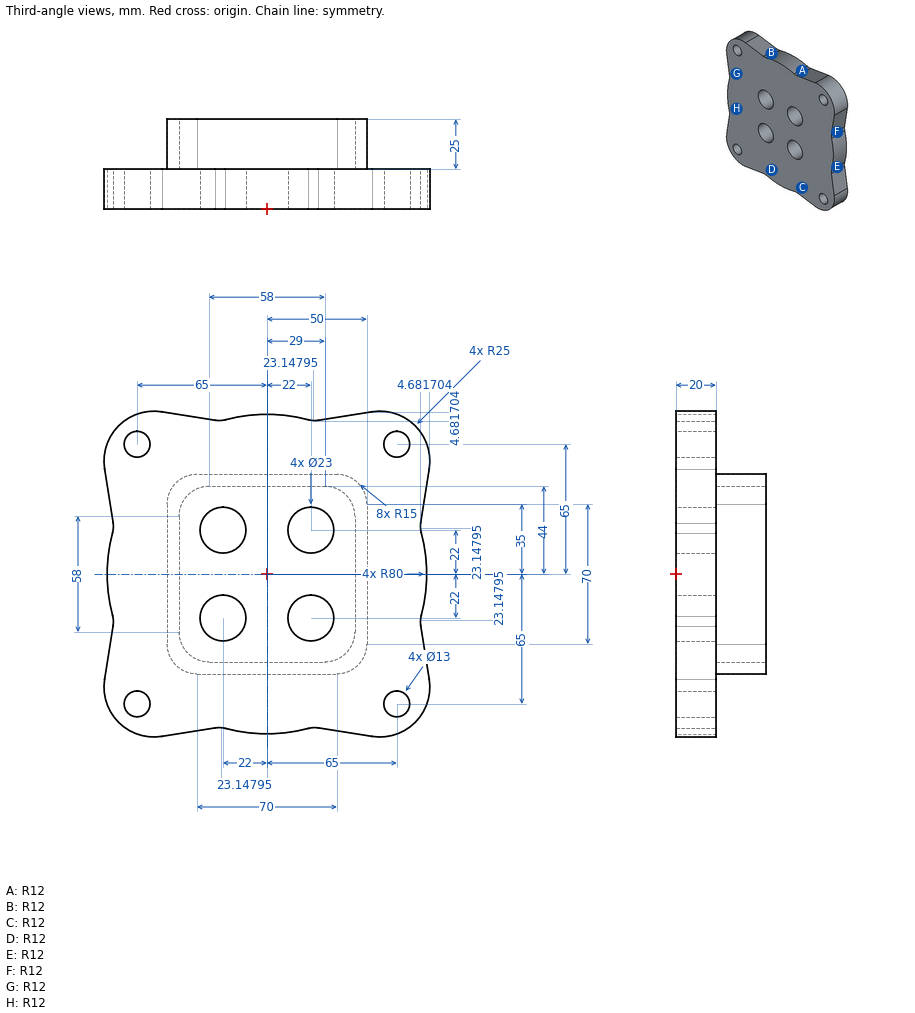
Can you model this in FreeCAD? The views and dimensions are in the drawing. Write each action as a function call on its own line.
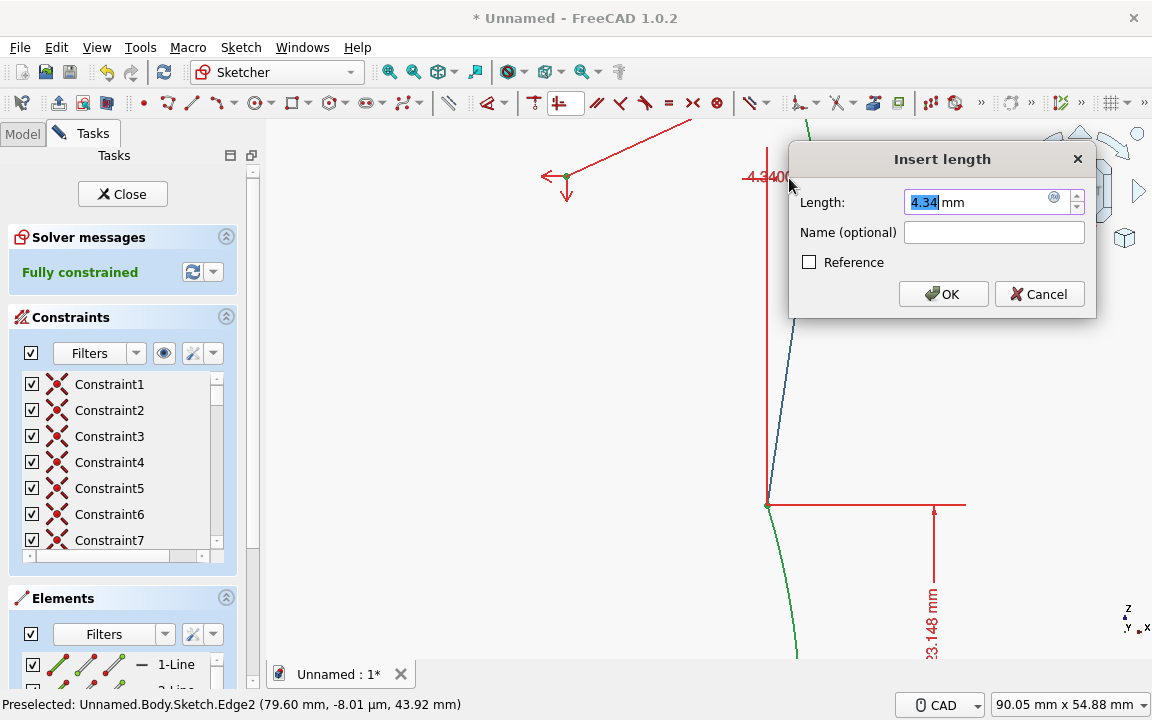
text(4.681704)
key(Return)
key(Escape)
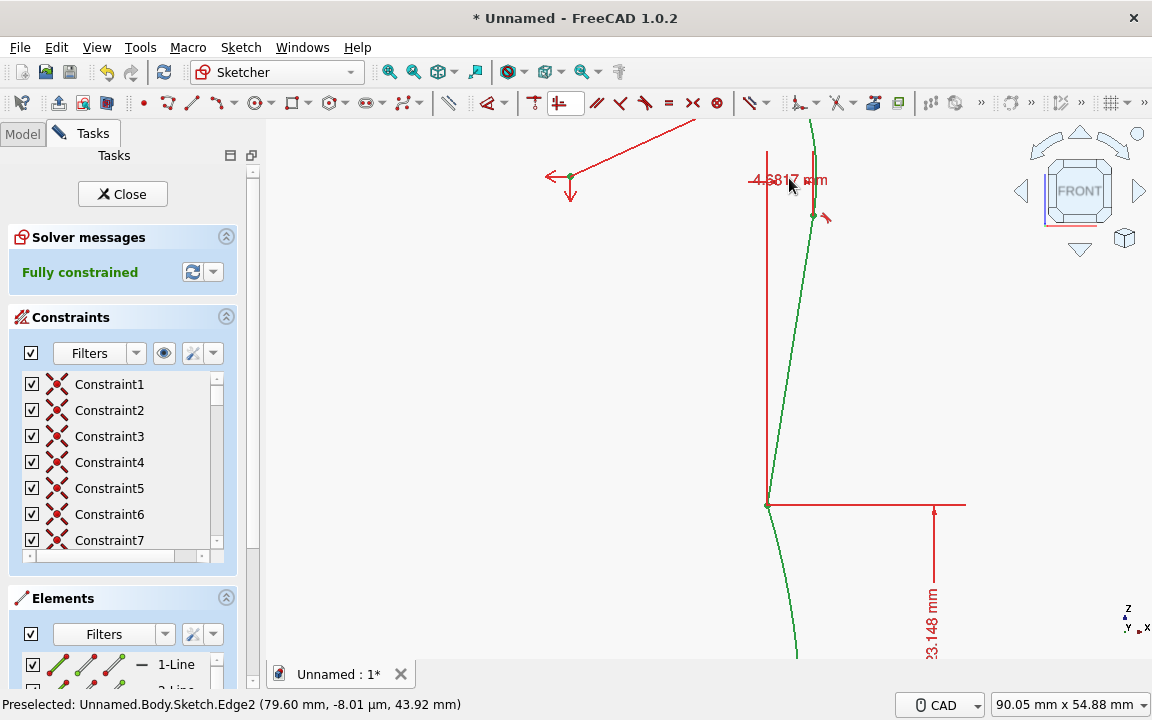
click(123, 194)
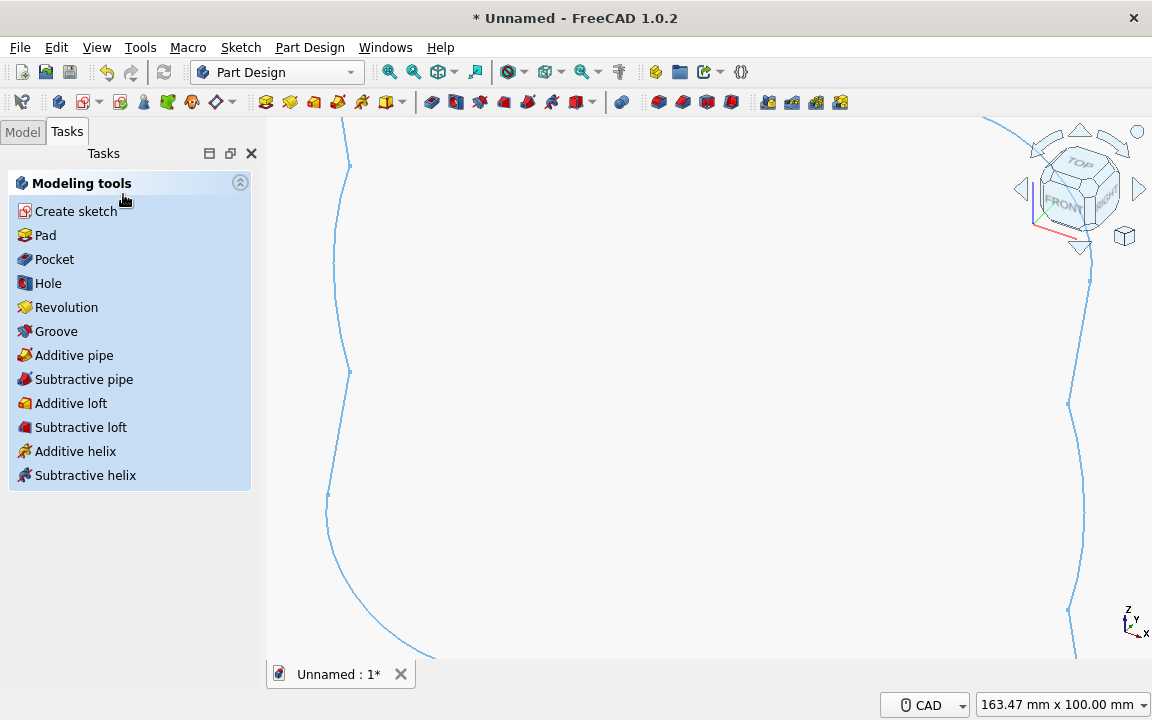
click(266, 102)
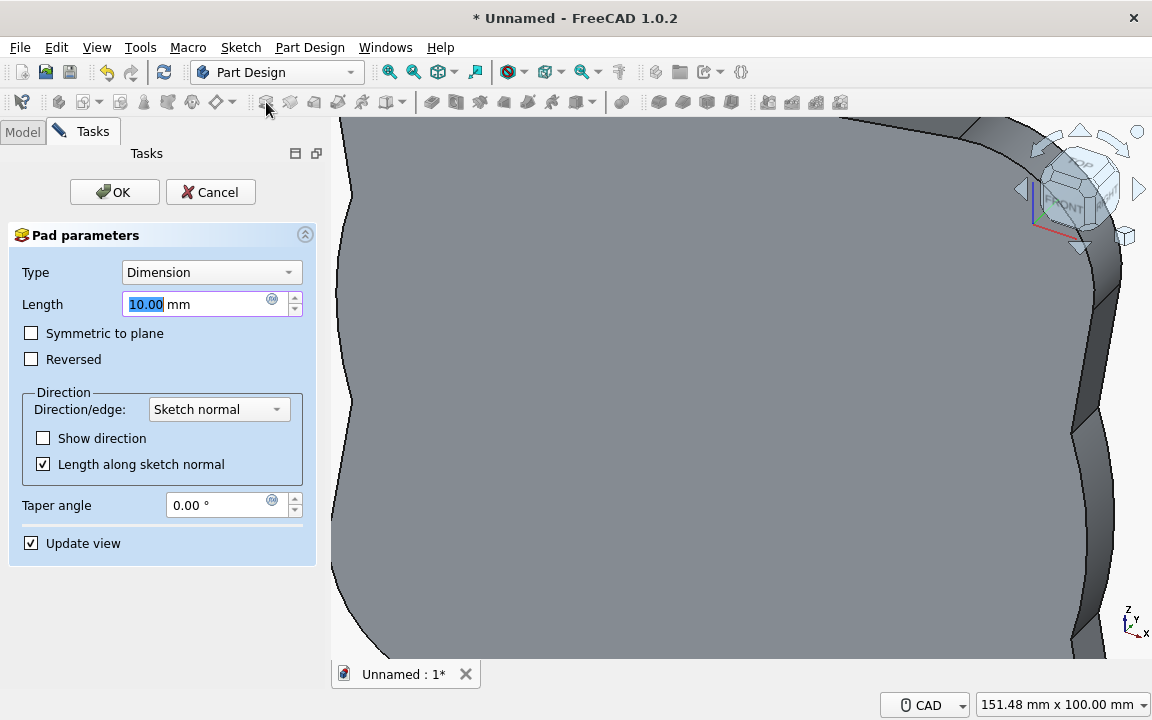
text(20)
key(Tab)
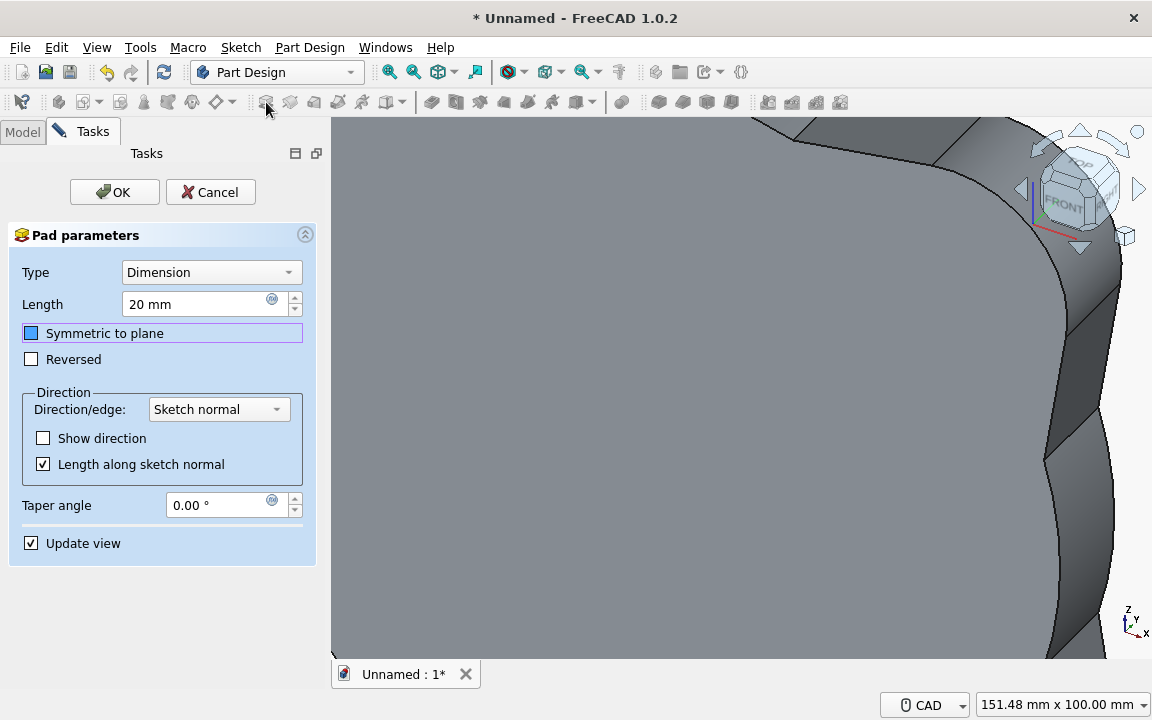
click(30, 359)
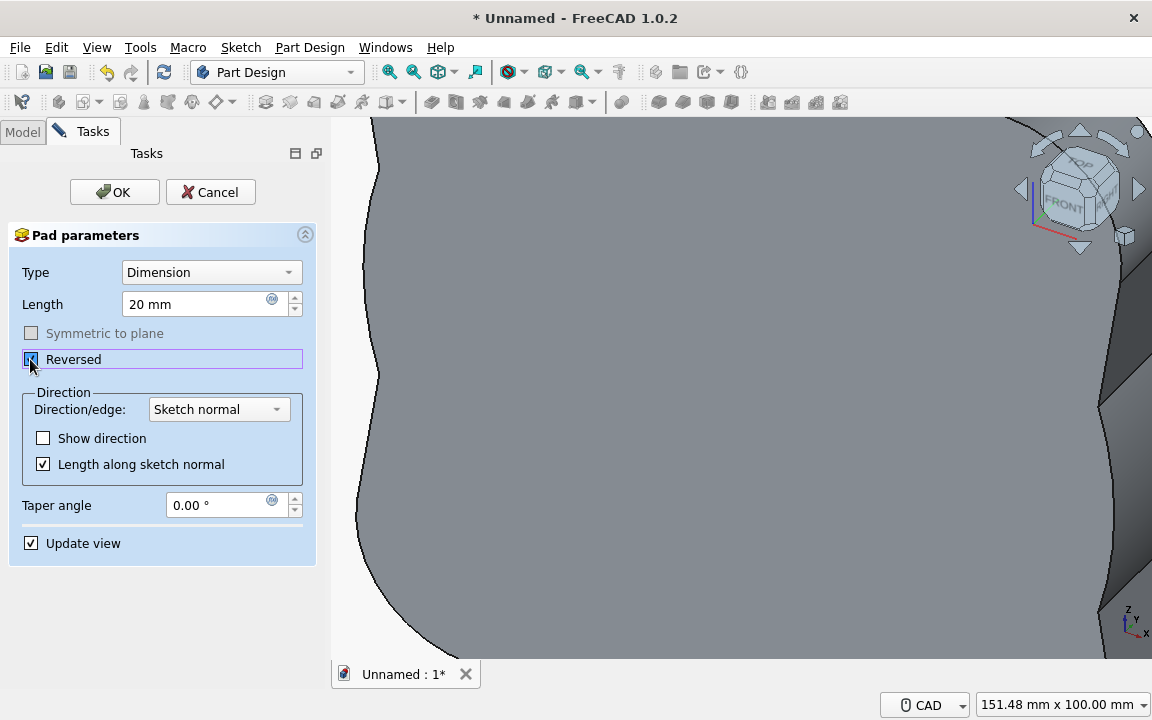
click(115, 192)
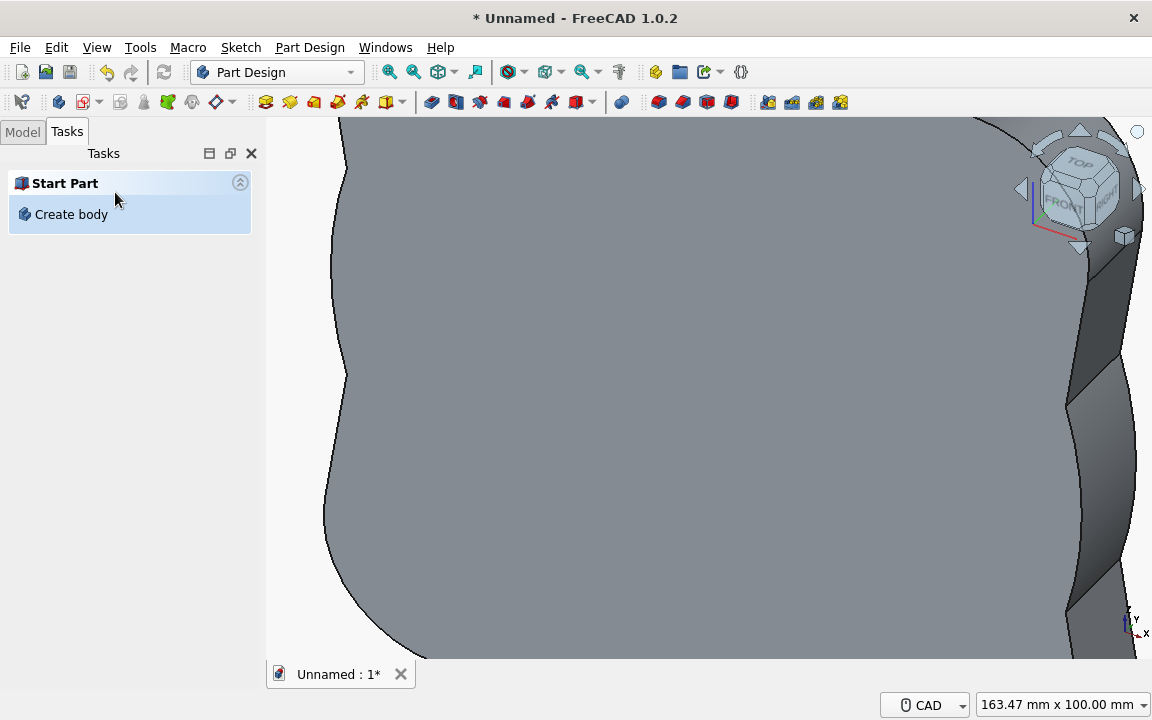
click(390, 72)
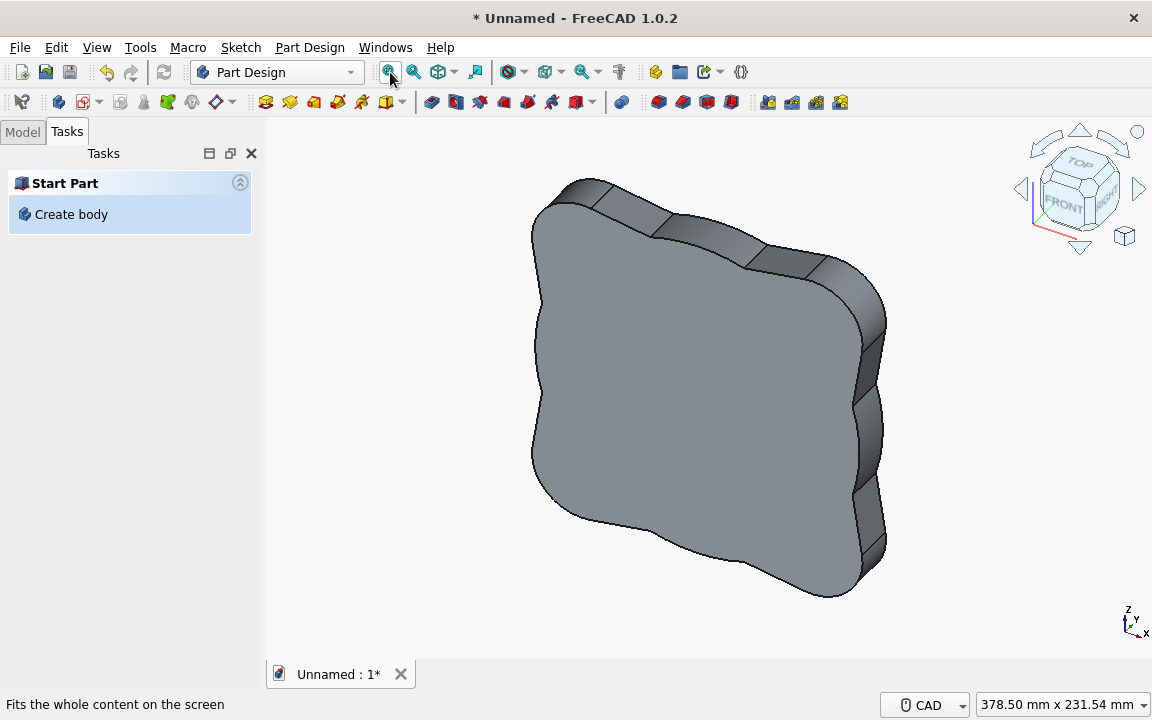
key(4)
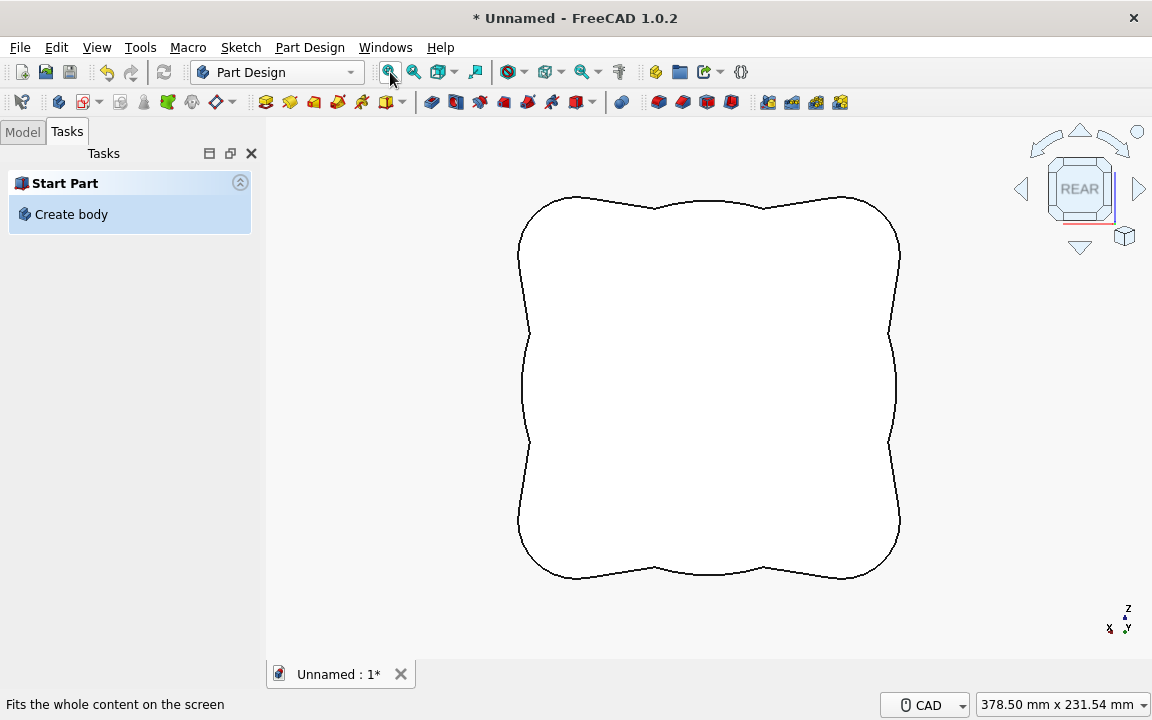
click(709, 387)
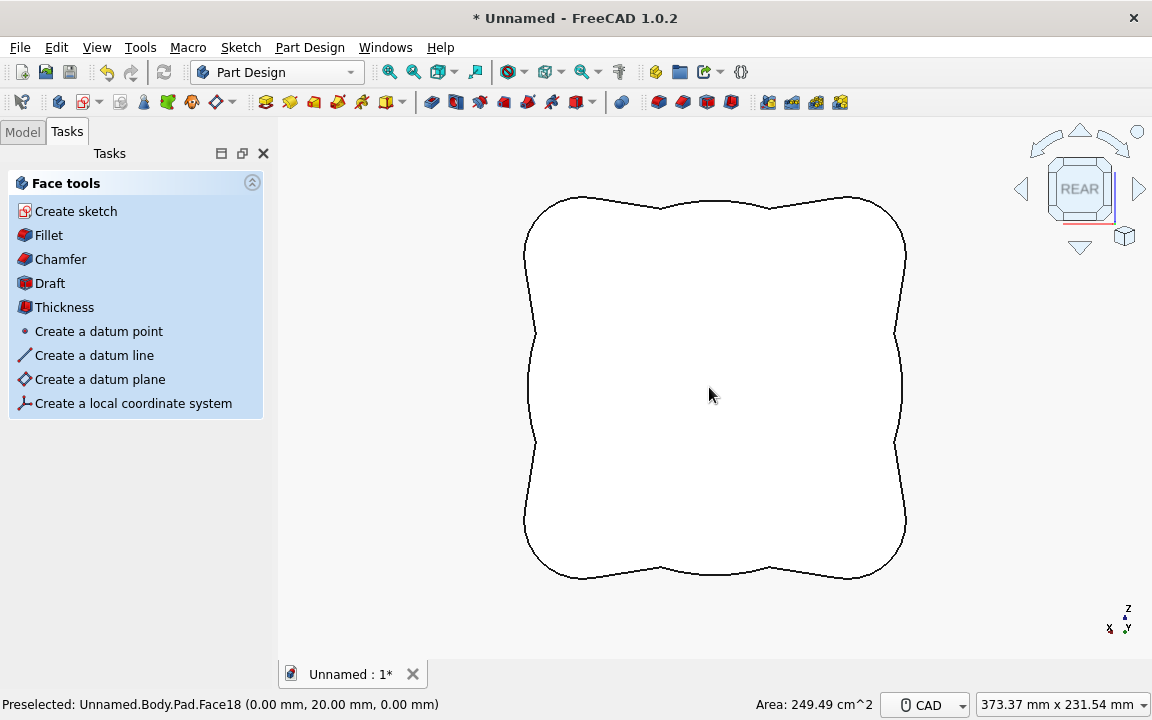
click(84, 102)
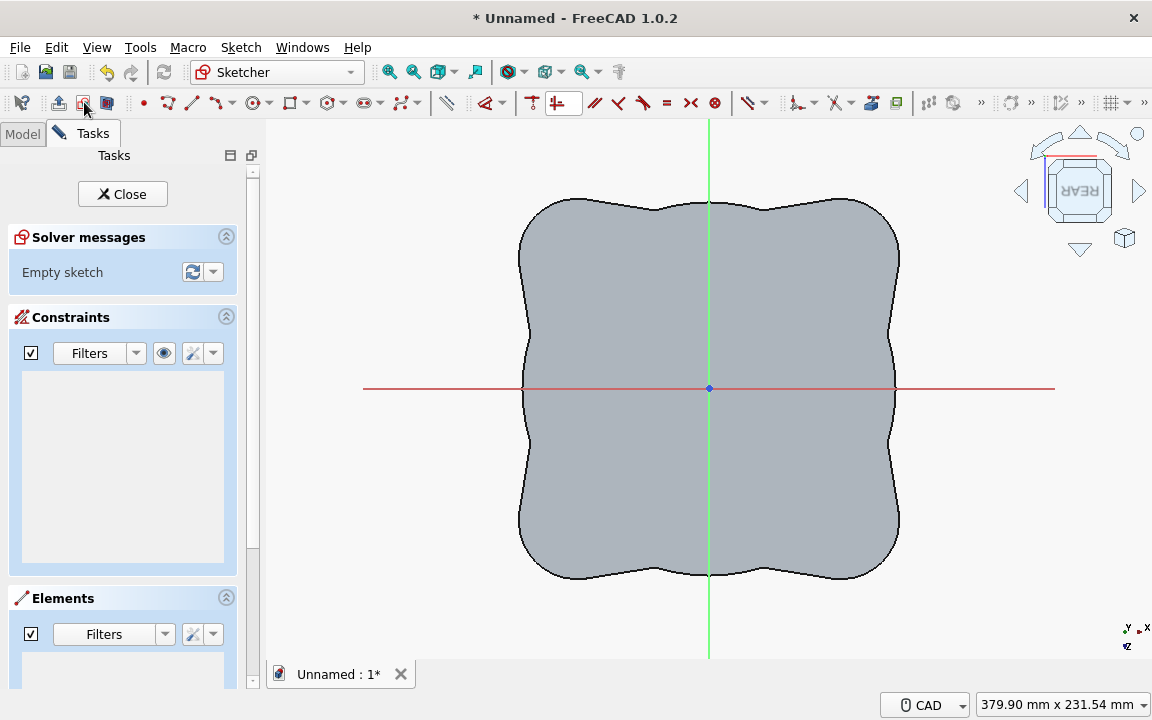
scroll(848, 389, up, 2)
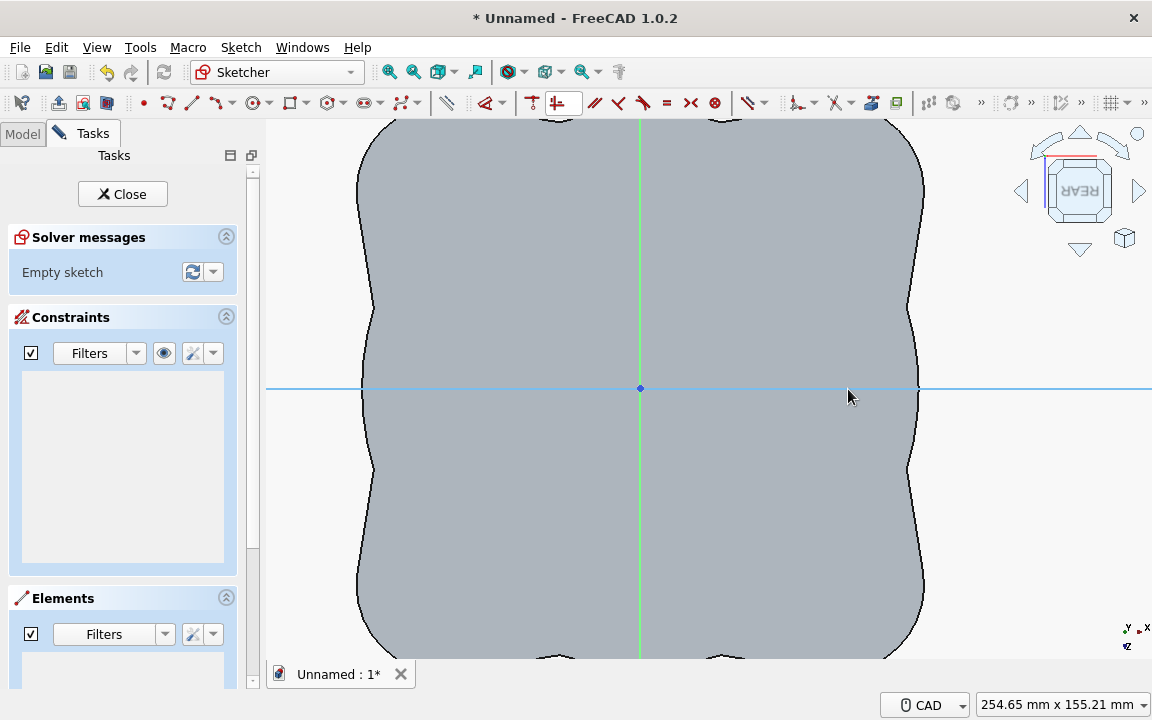
click(192, 104)